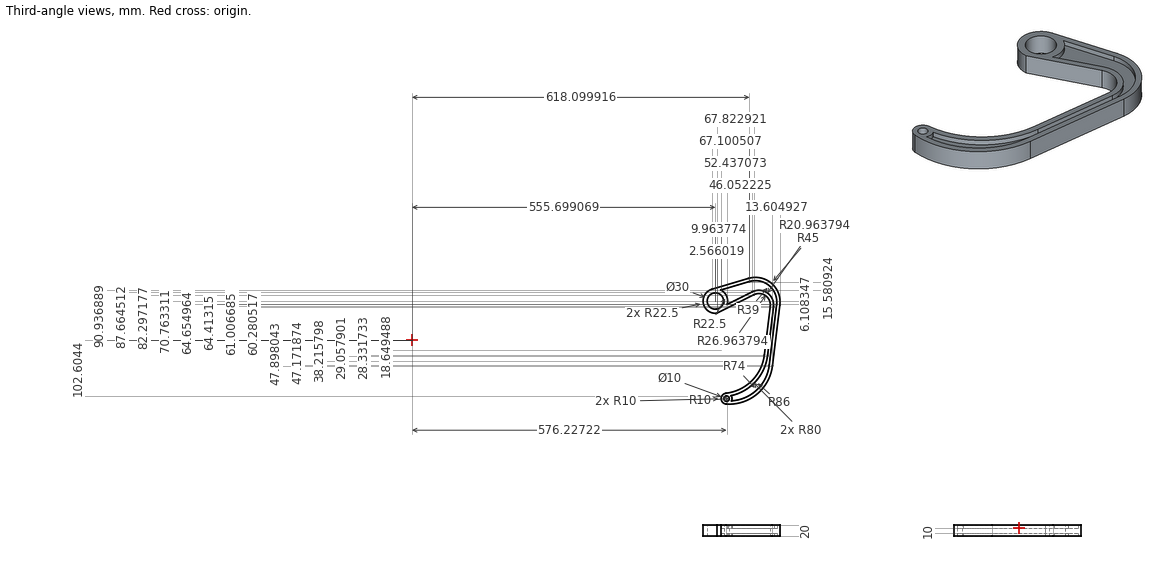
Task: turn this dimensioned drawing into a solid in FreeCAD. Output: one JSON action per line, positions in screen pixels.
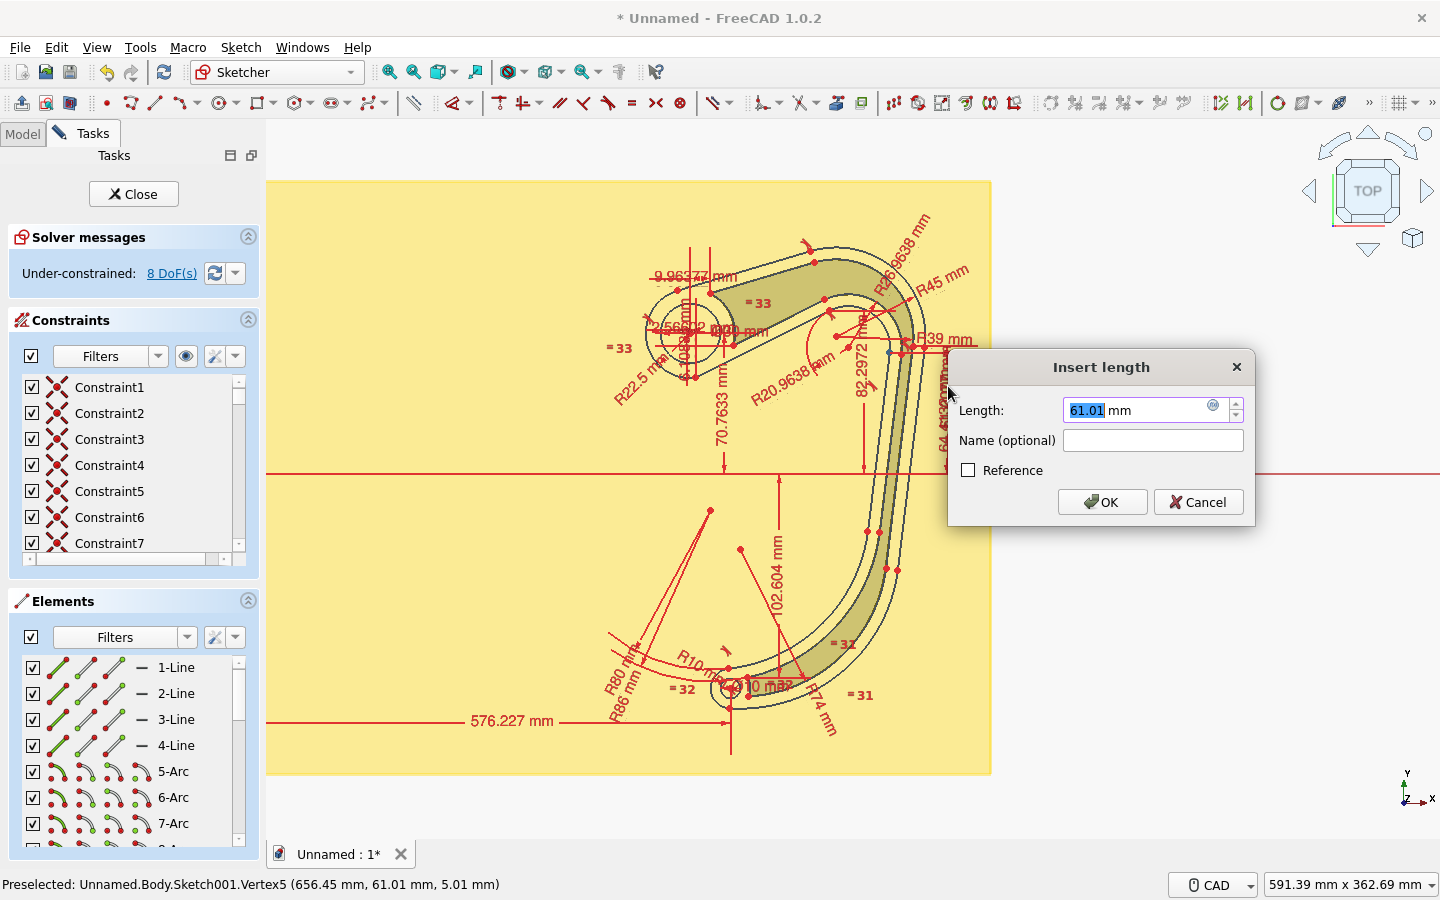
{"action": "type", "text": "61.006685"}
{"action": "key", "text": "Return"}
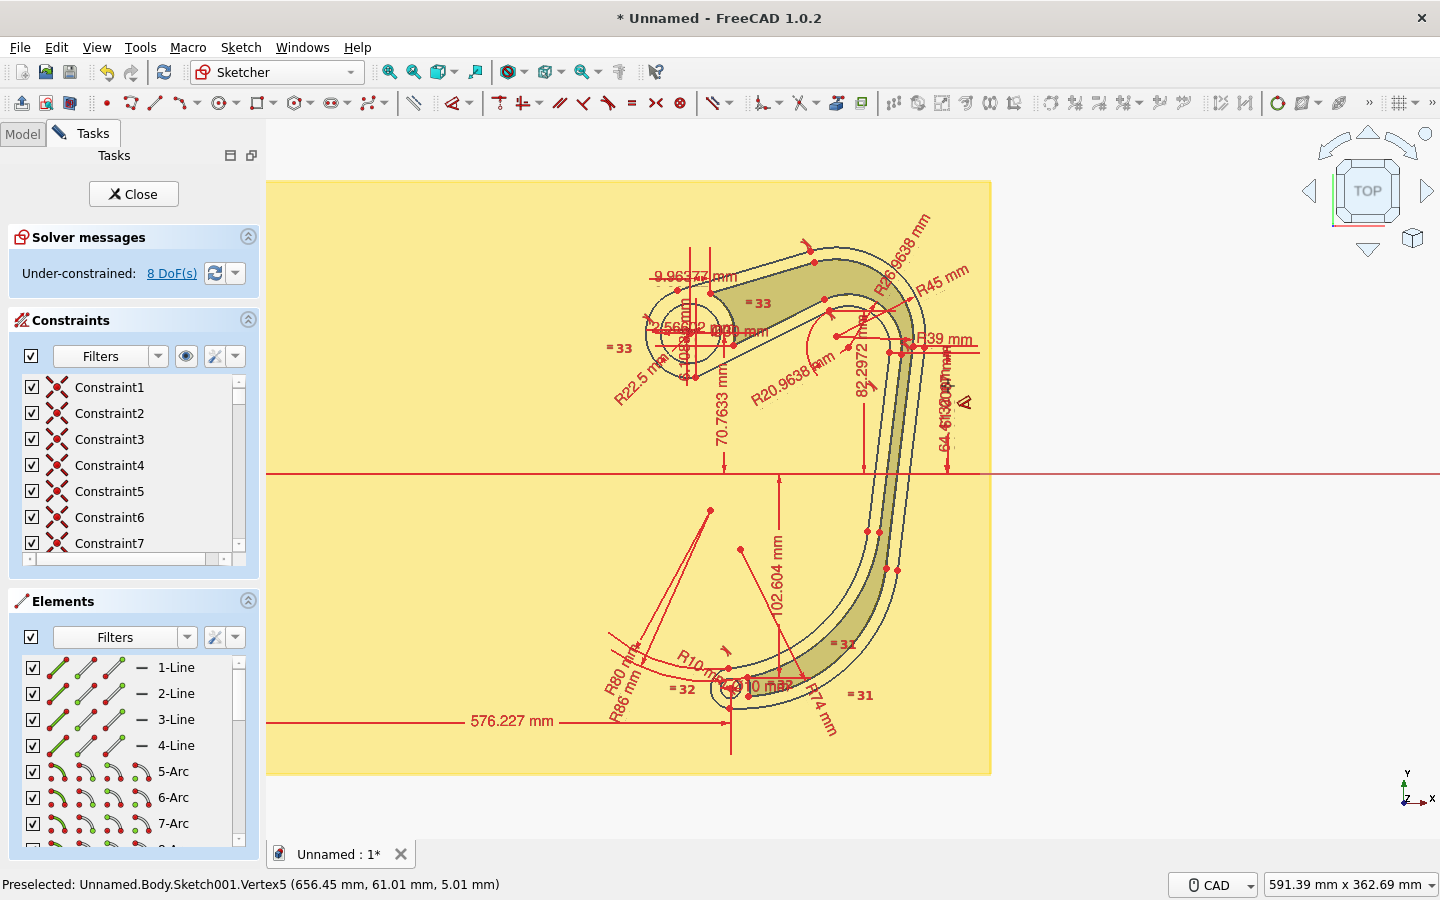
{"action": "left_click", "coordinate": [868, 531]}
{"action": "left_click", "coordinate": [926, 503]}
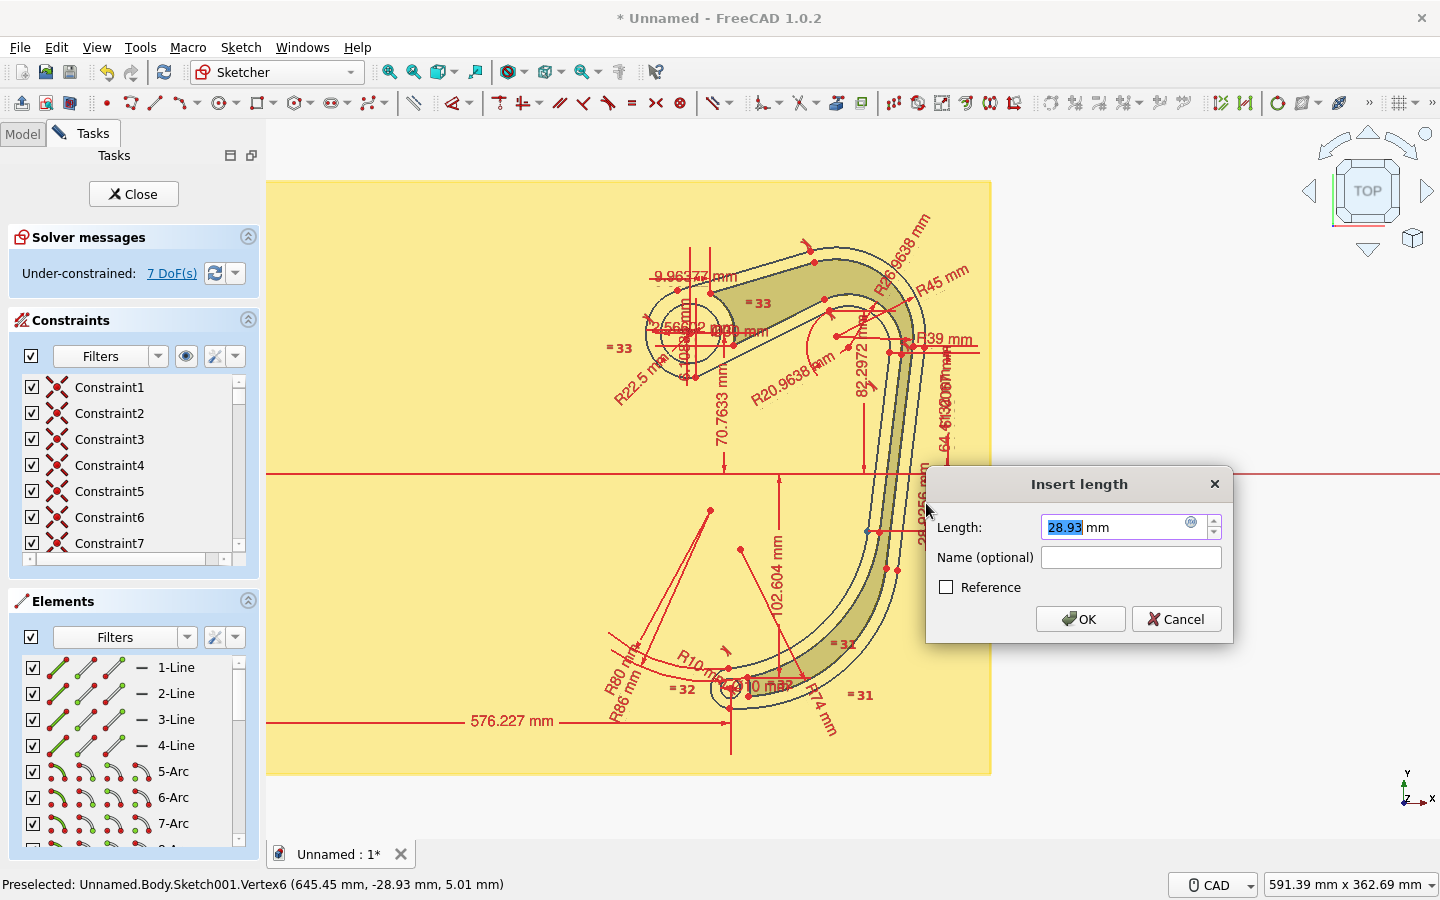
{"action": "type", "text": "28.331733"}
{"action": "key", "text": "Return"}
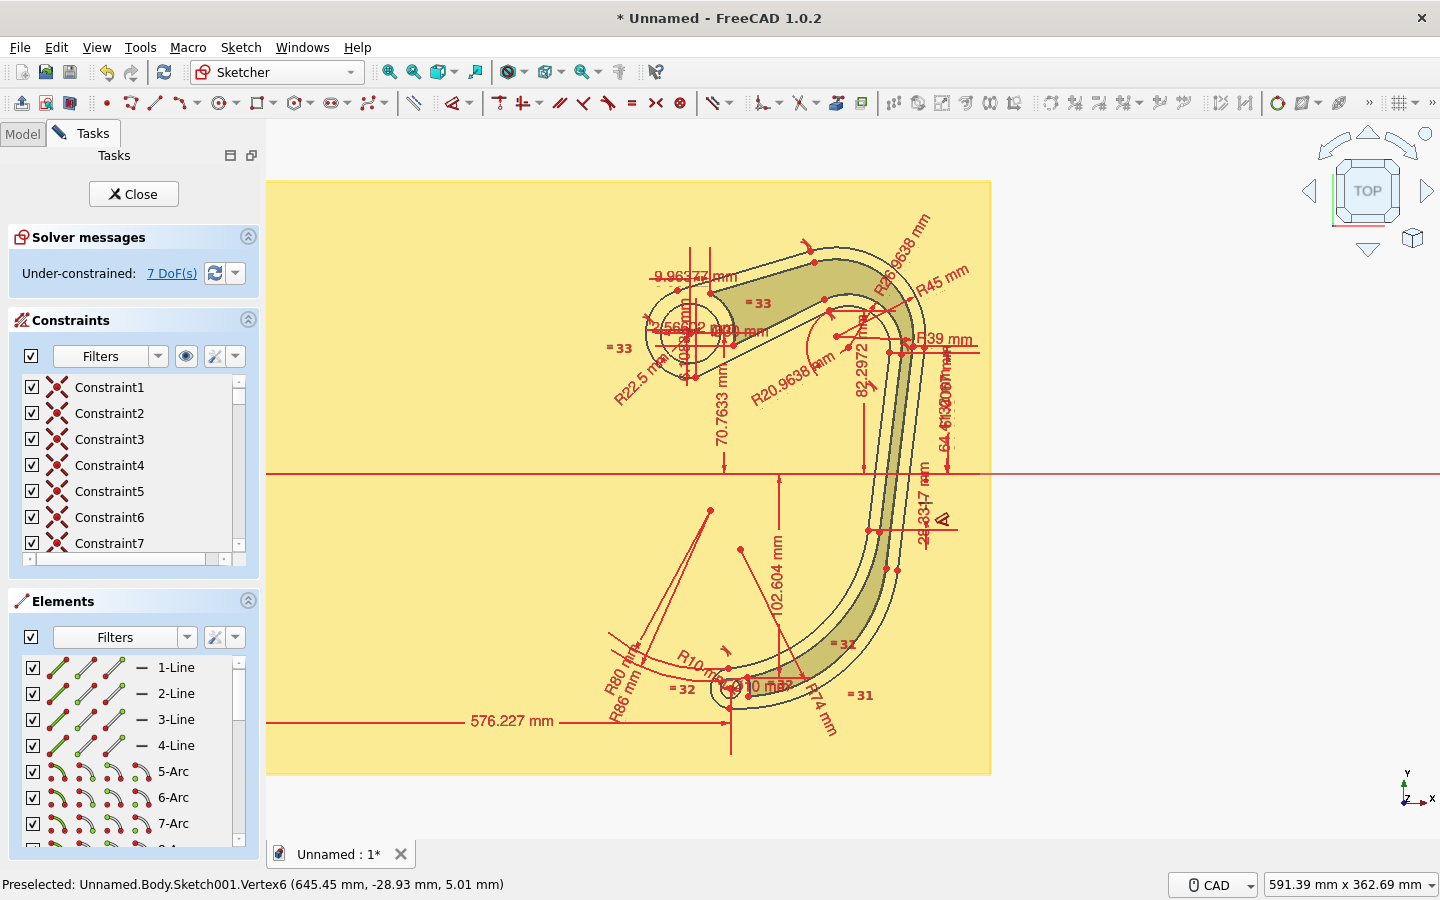
{"action": "left_click", "coordinate": [898, 570]}
{"action": "left_click", "coordinate": [932, 544]}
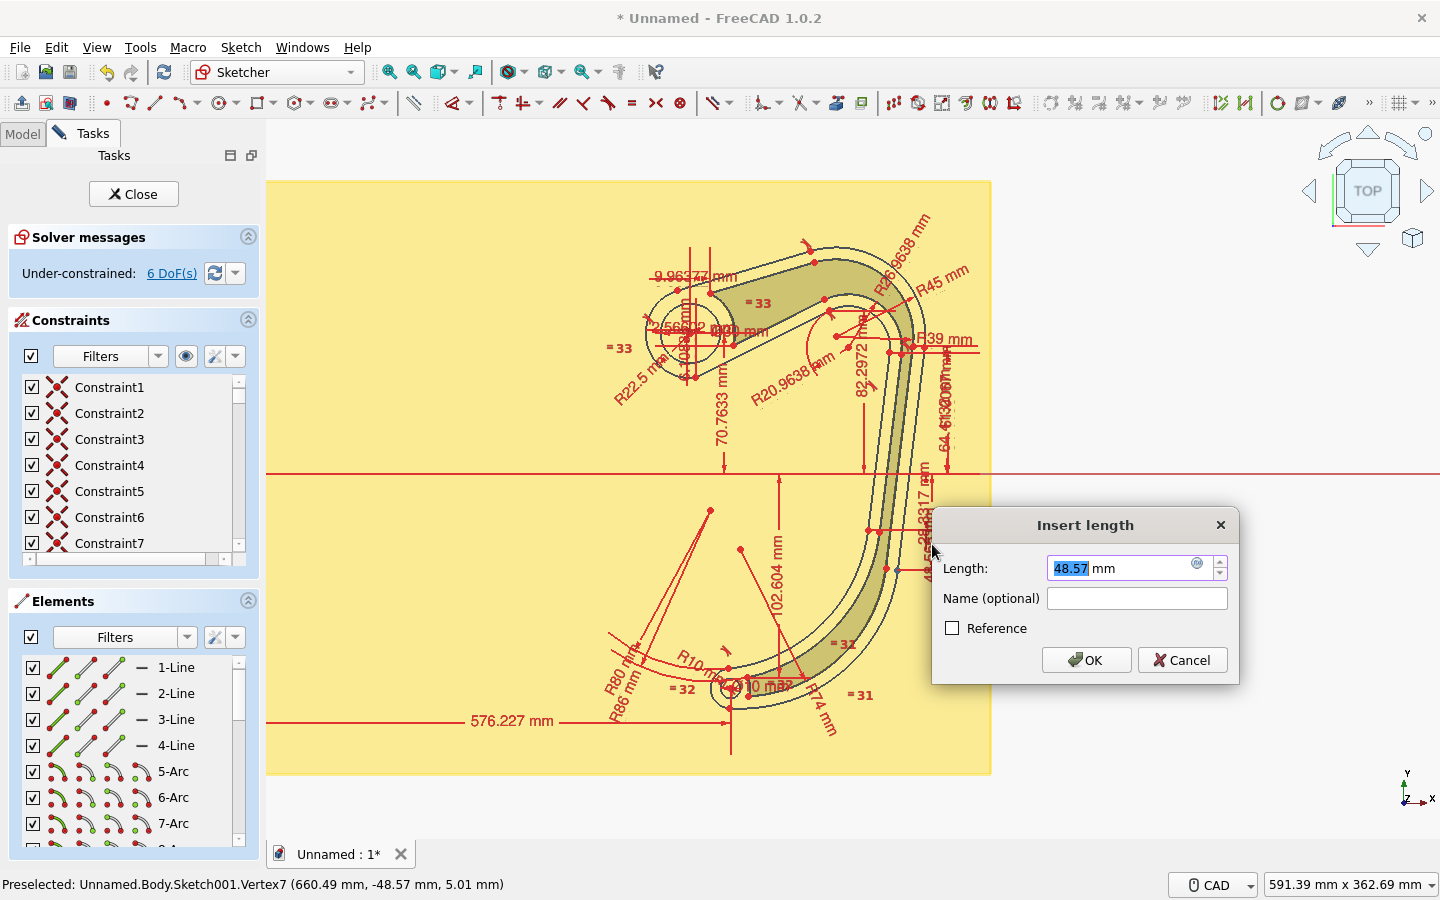
{"action": "type", "text": "47.898043"}
{"action": "key", "text": "Return"}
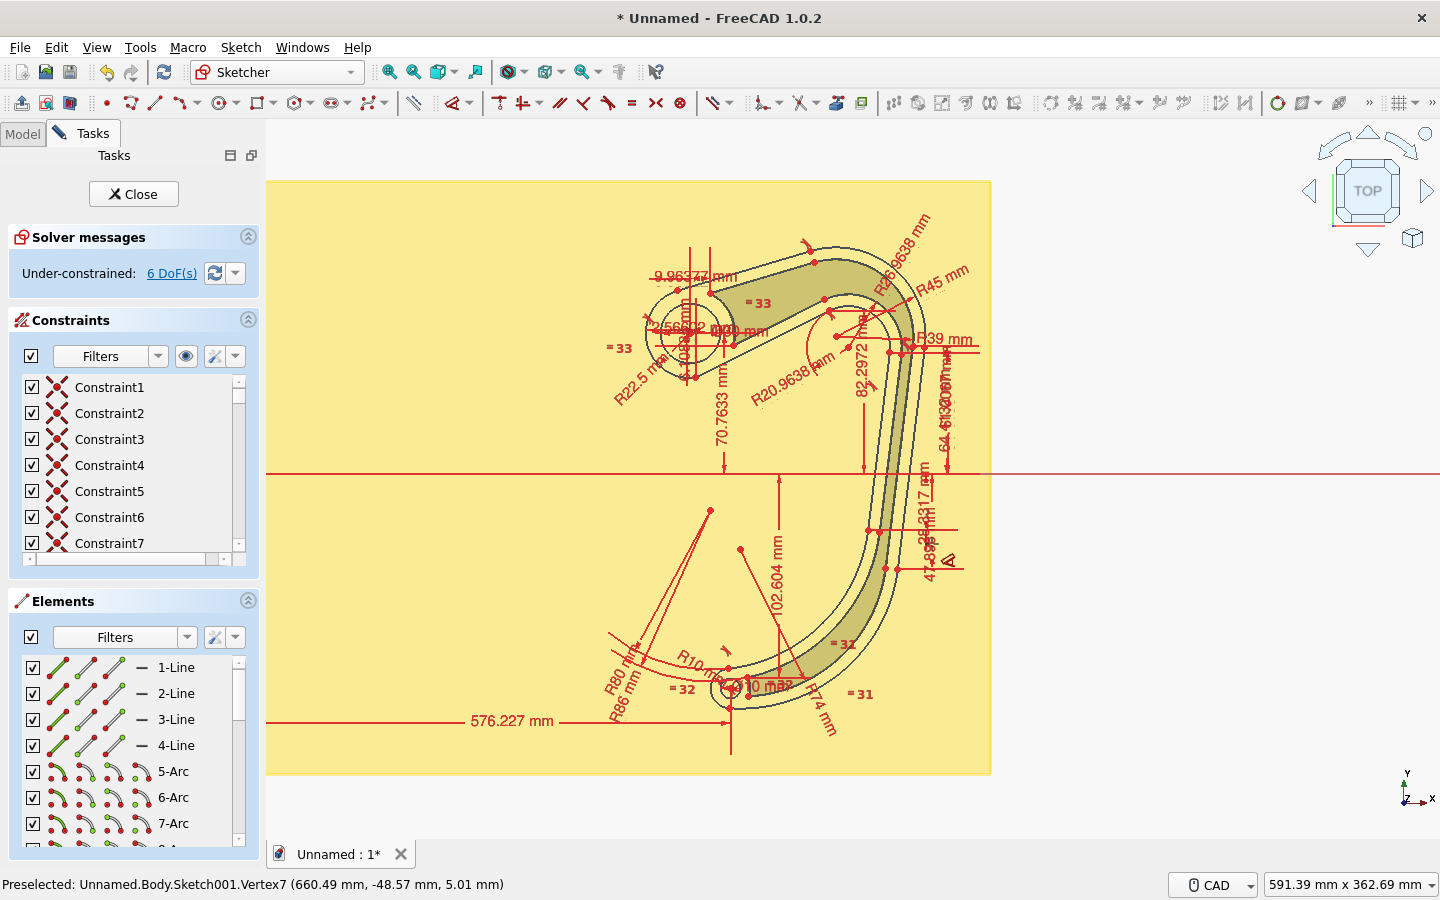
{"action": "left_click", "coordinate": [886, 568]}
{"action": "left_click", "coordinate": [1016, 521]}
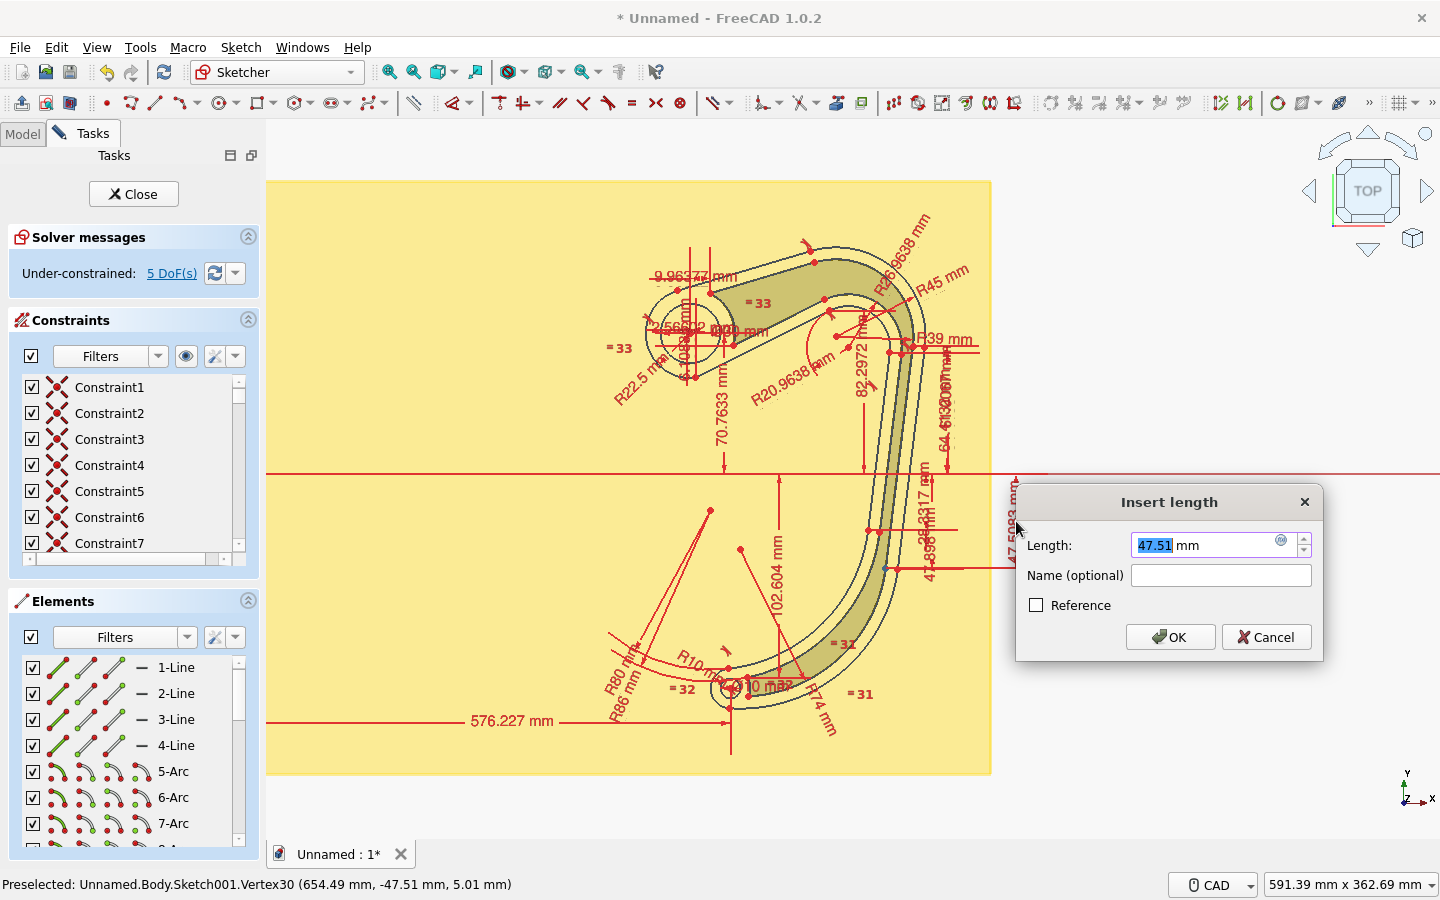
{"action": "type", "text": "47.171874"}
{"action": "key", "text": "Return"}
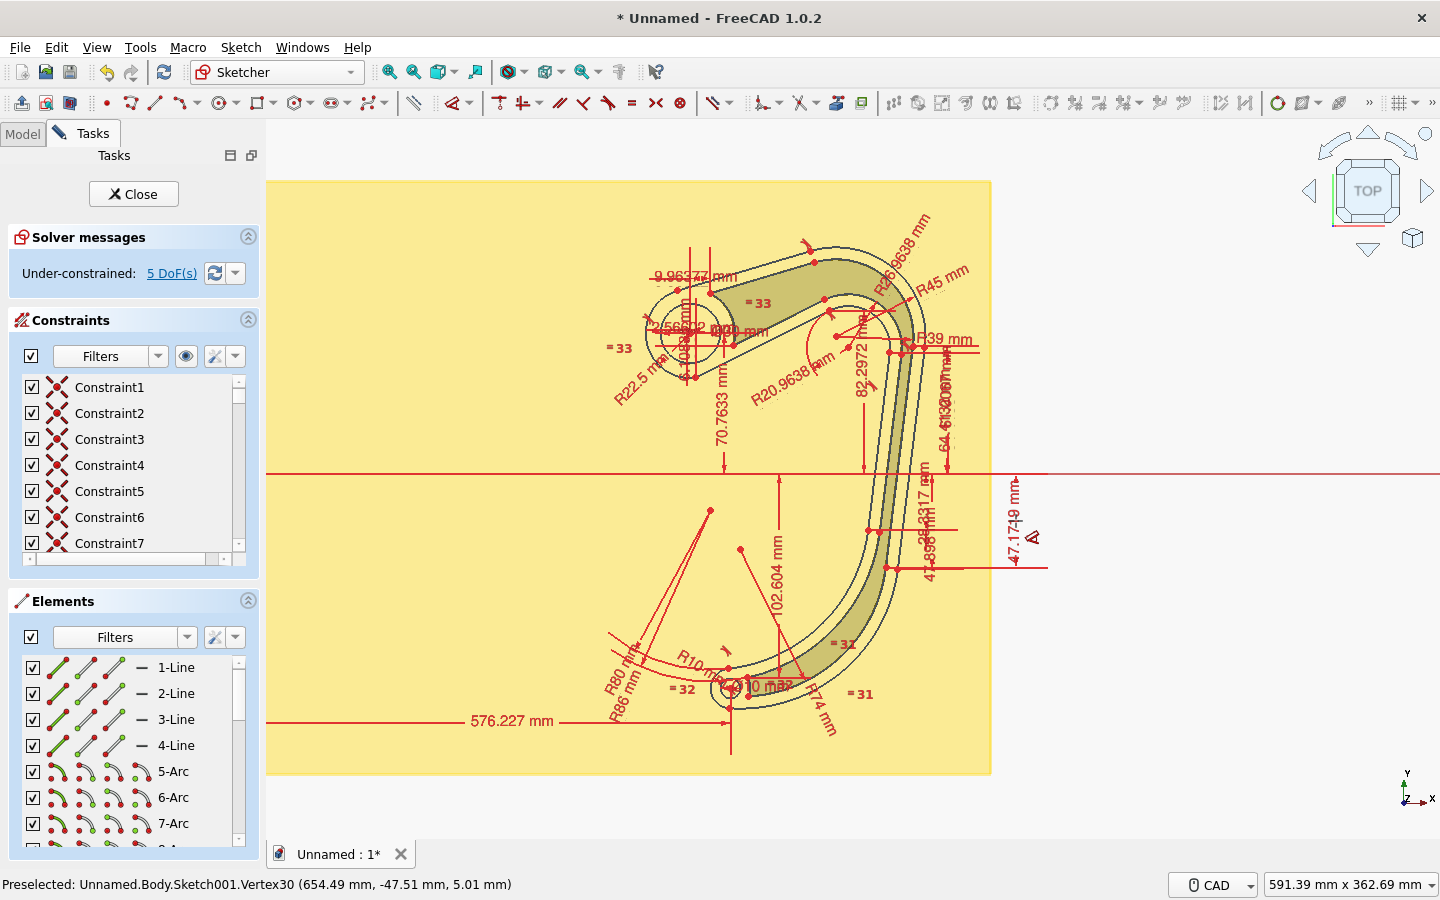
{"action": "left_click", "coordinate": [880, 532]}
{"action": "left_click", "coordinate": [938, 523]}